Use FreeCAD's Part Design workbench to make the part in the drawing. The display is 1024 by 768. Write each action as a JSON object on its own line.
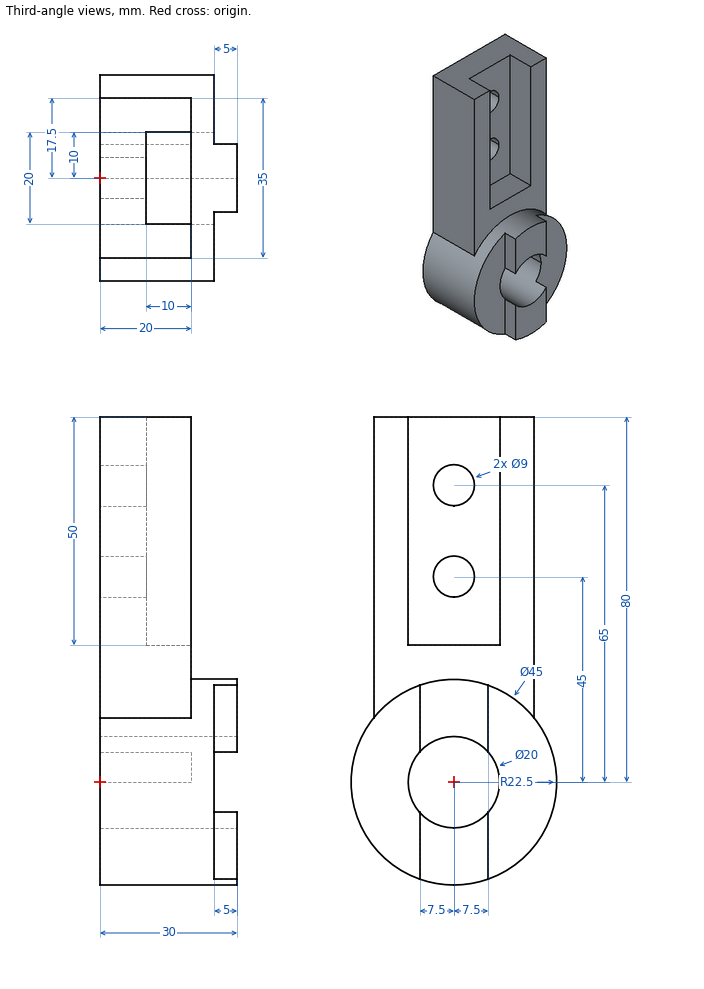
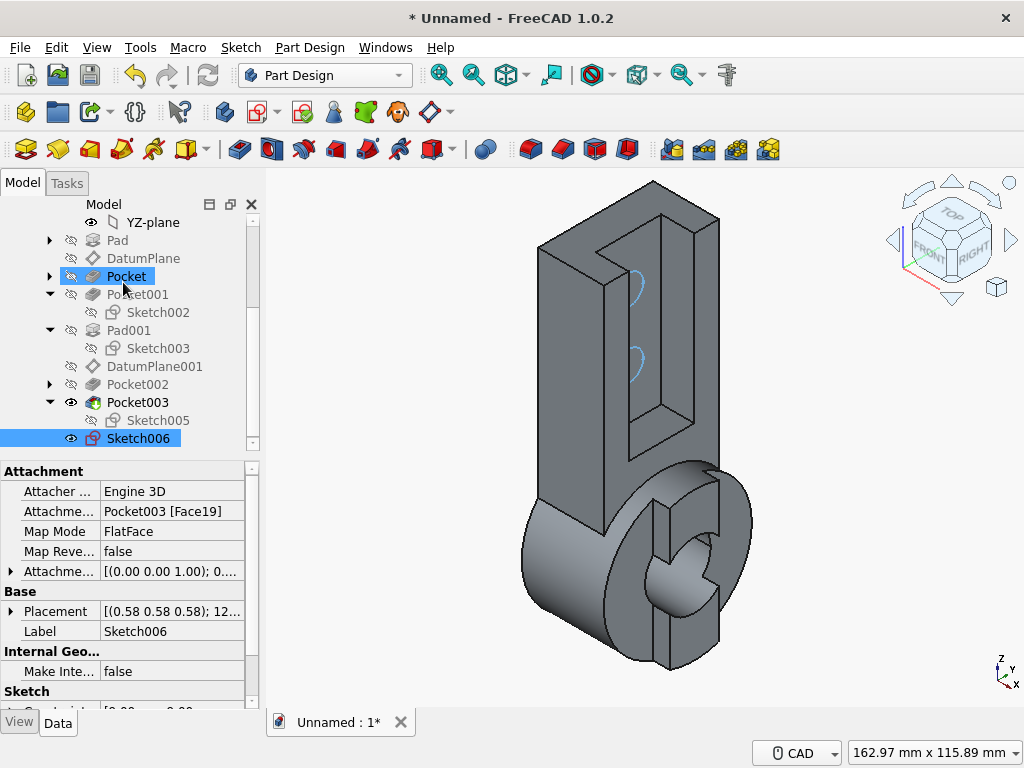
{"action": "left_click", "coordinate": [240, 150]}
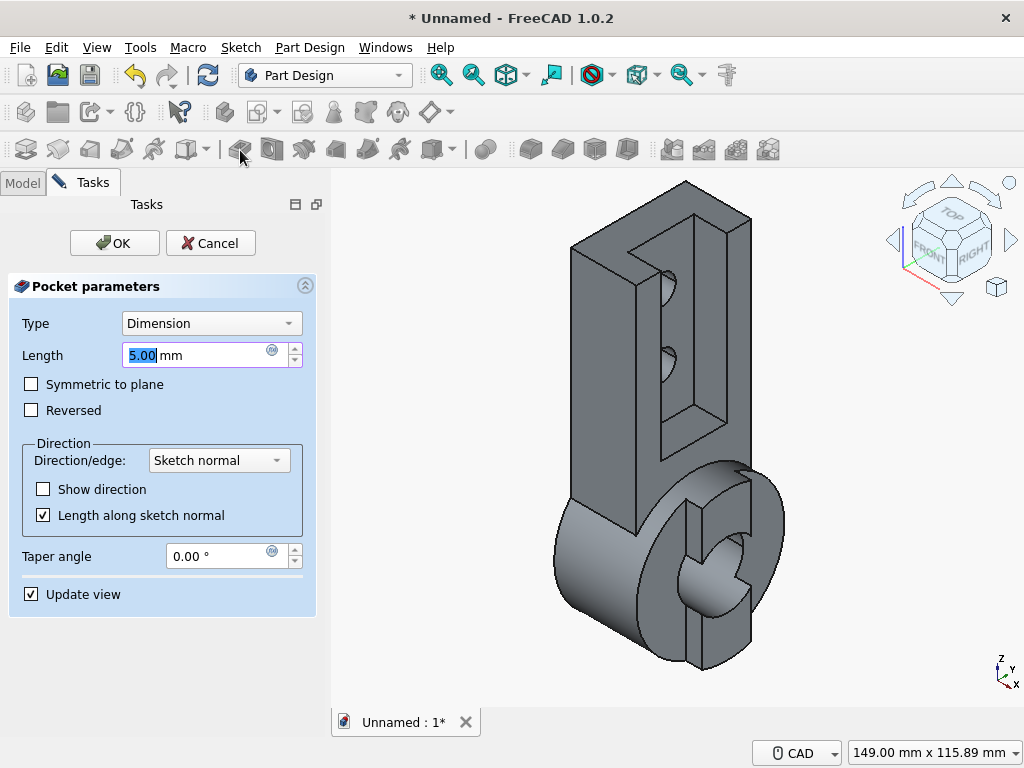
{"action": "left_click", "coordinate": [212, 324]}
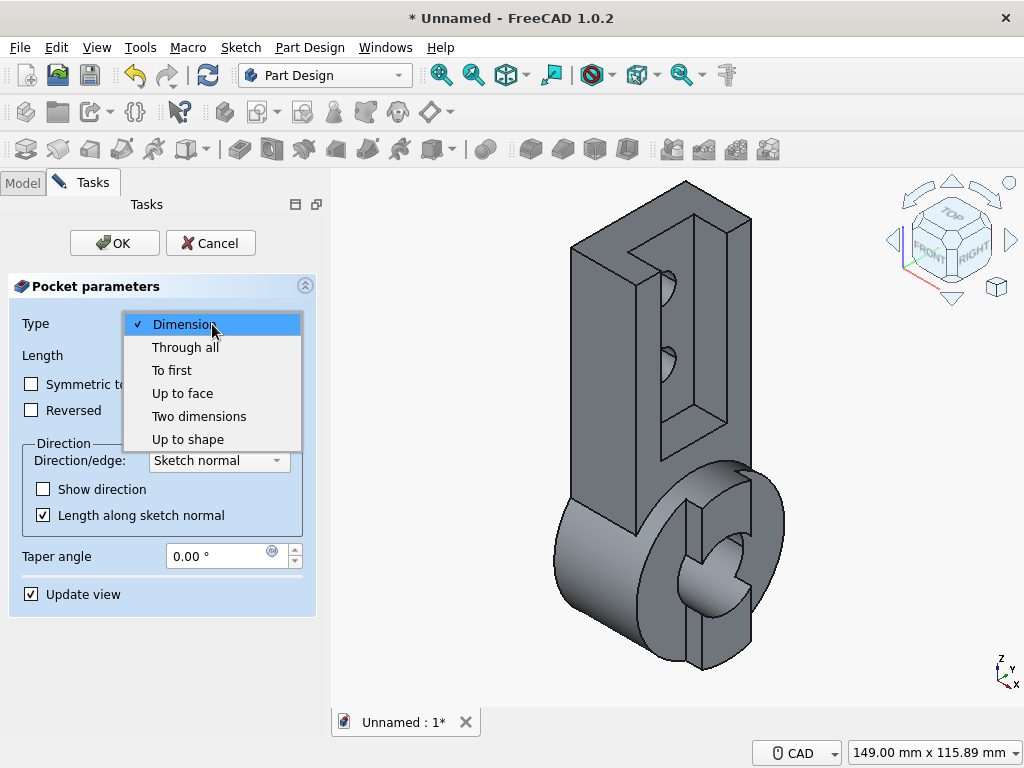
{"action": "left_click", "coordinate": [212, 348]}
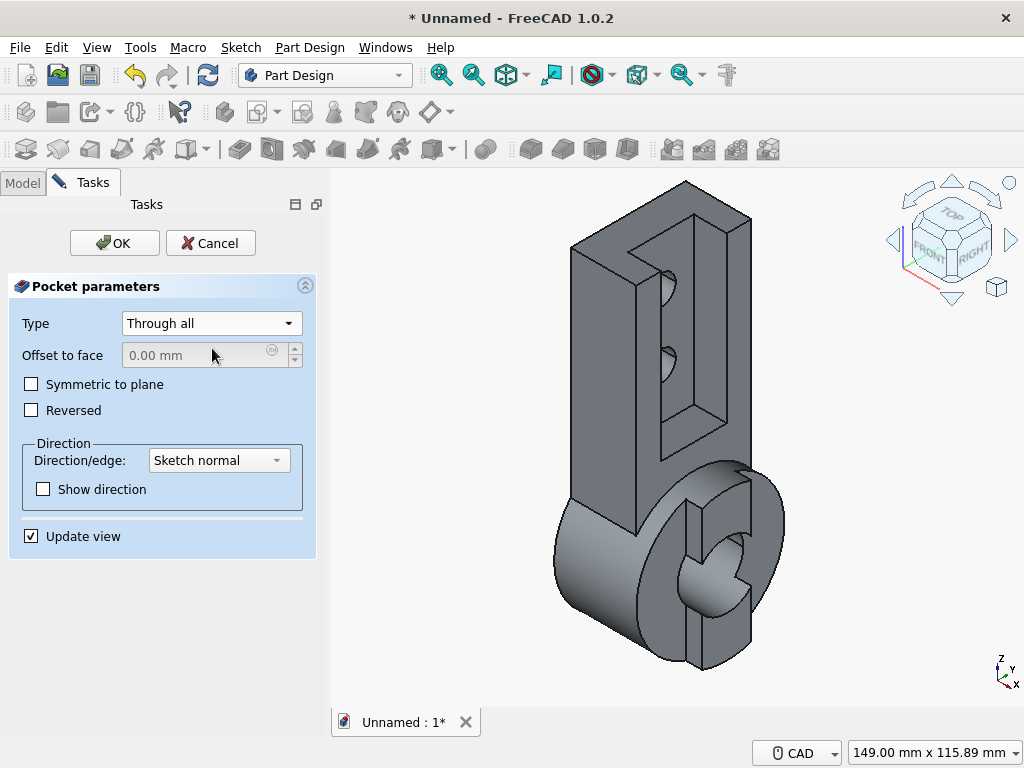
{"action": "left_click", "coordinate": [115, 243]}